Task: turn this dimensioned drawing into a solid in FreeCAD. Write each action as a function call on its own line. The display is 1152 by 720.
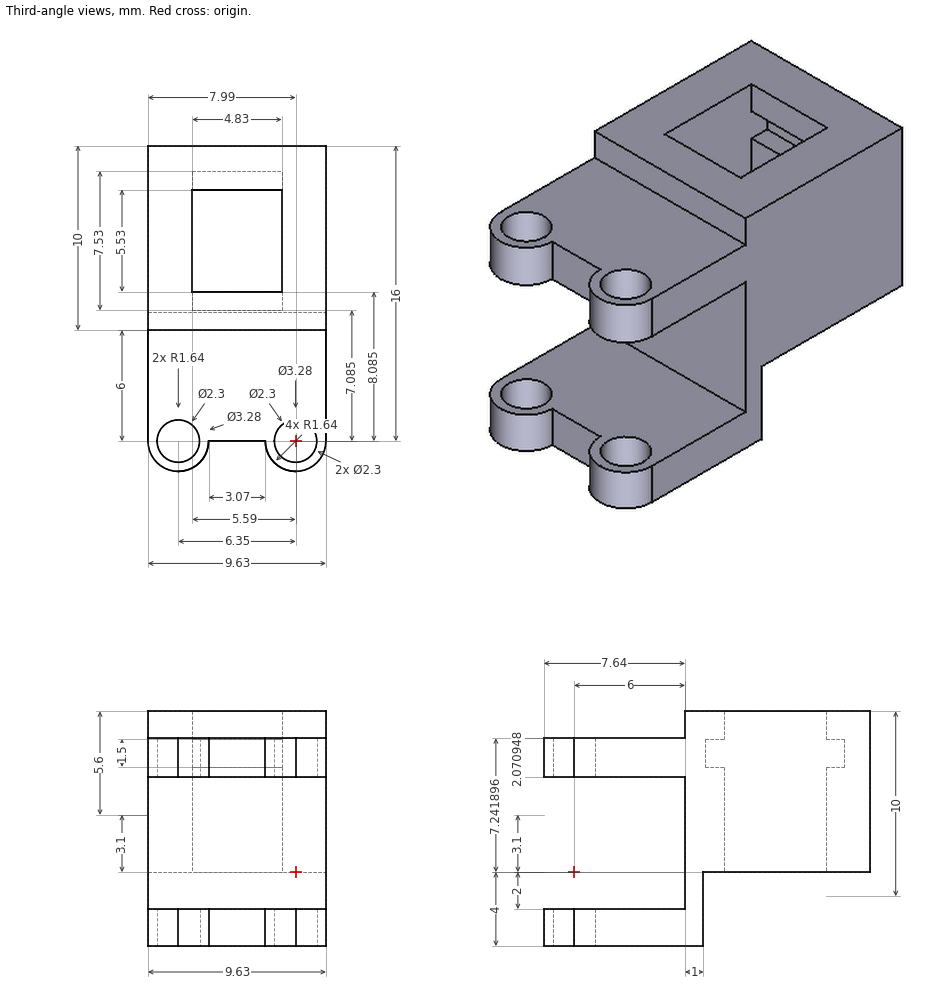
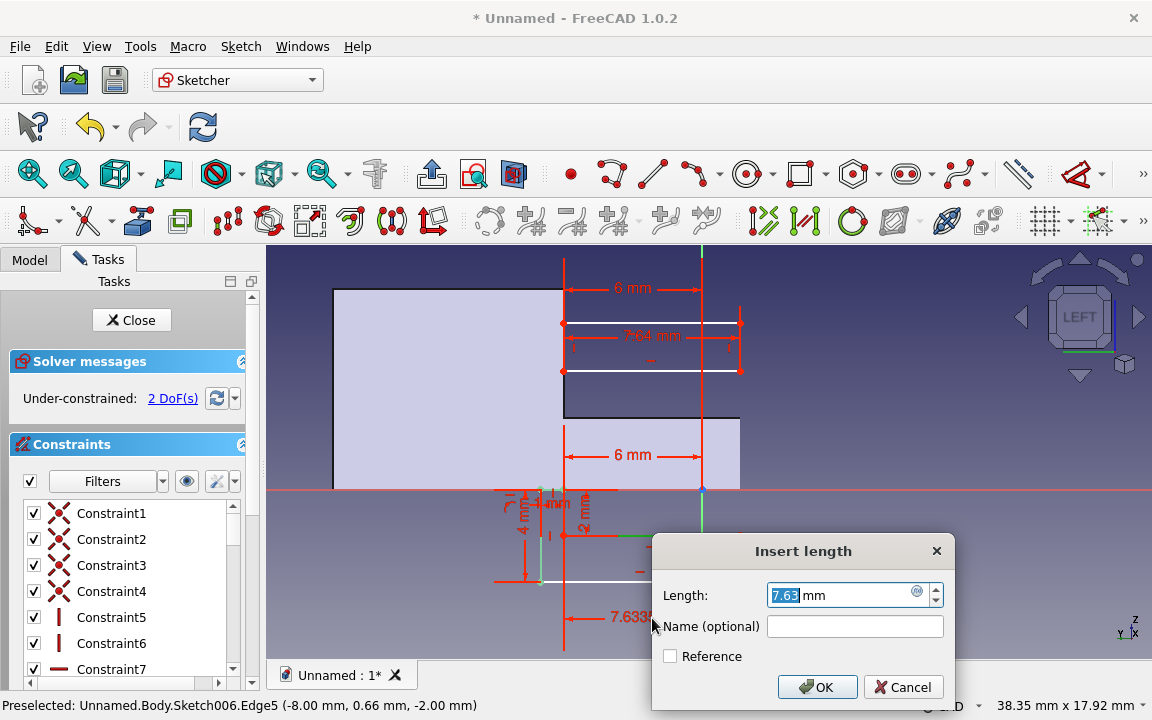
text(7.64)
key(Return)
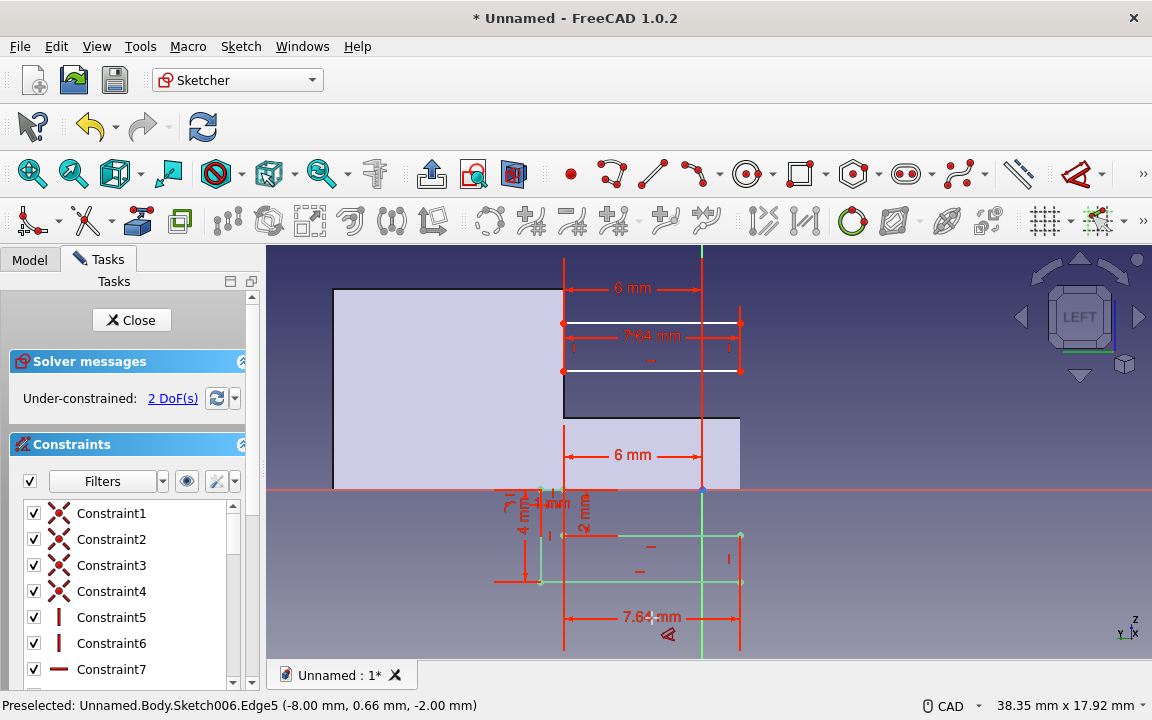
click(564, 337)
click(530, 347)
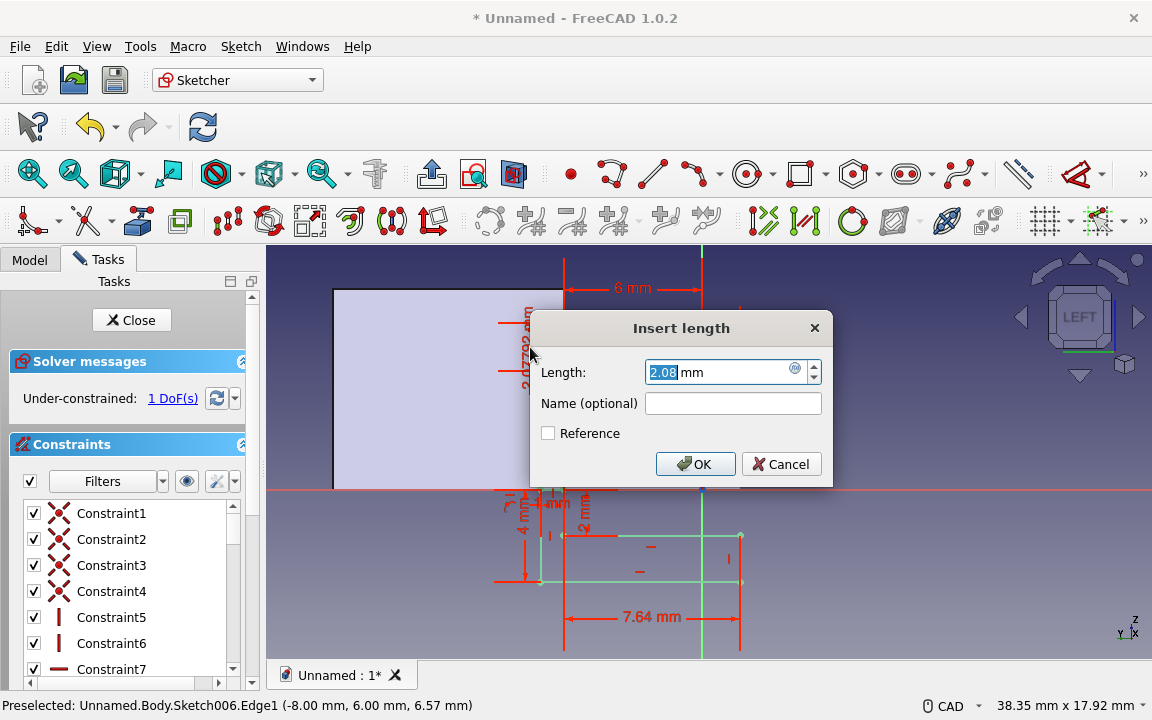
text(2.070948)
key(Return)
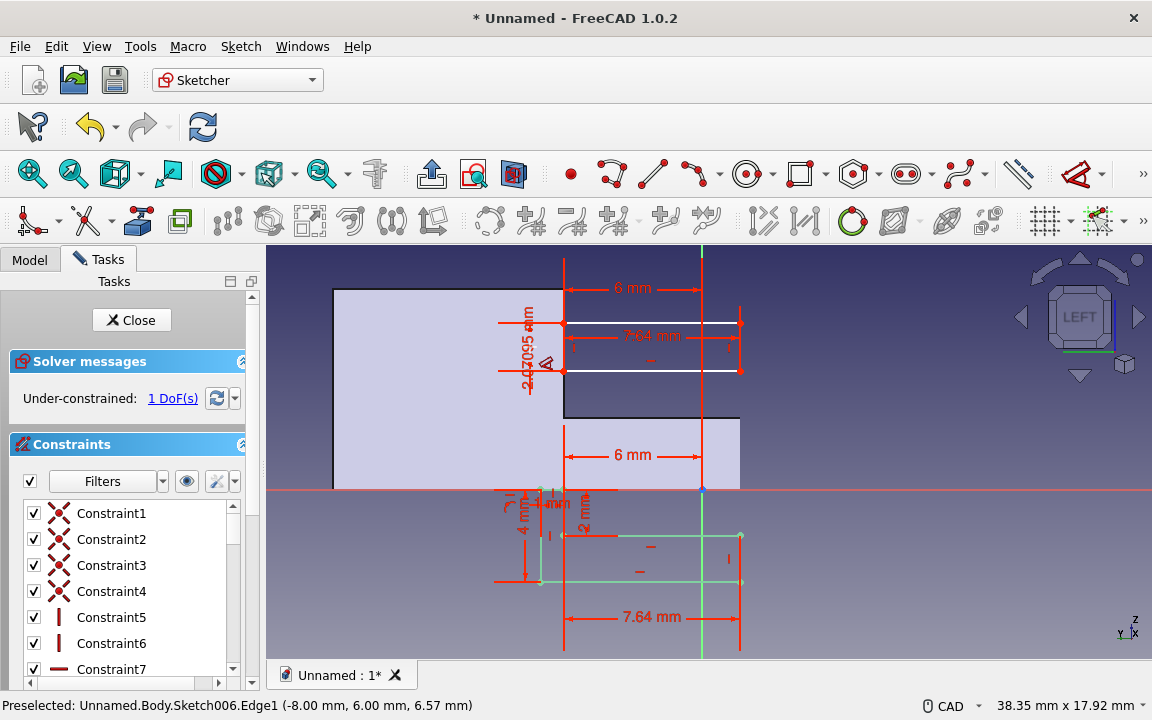
click(564, 323)
click(530, 406)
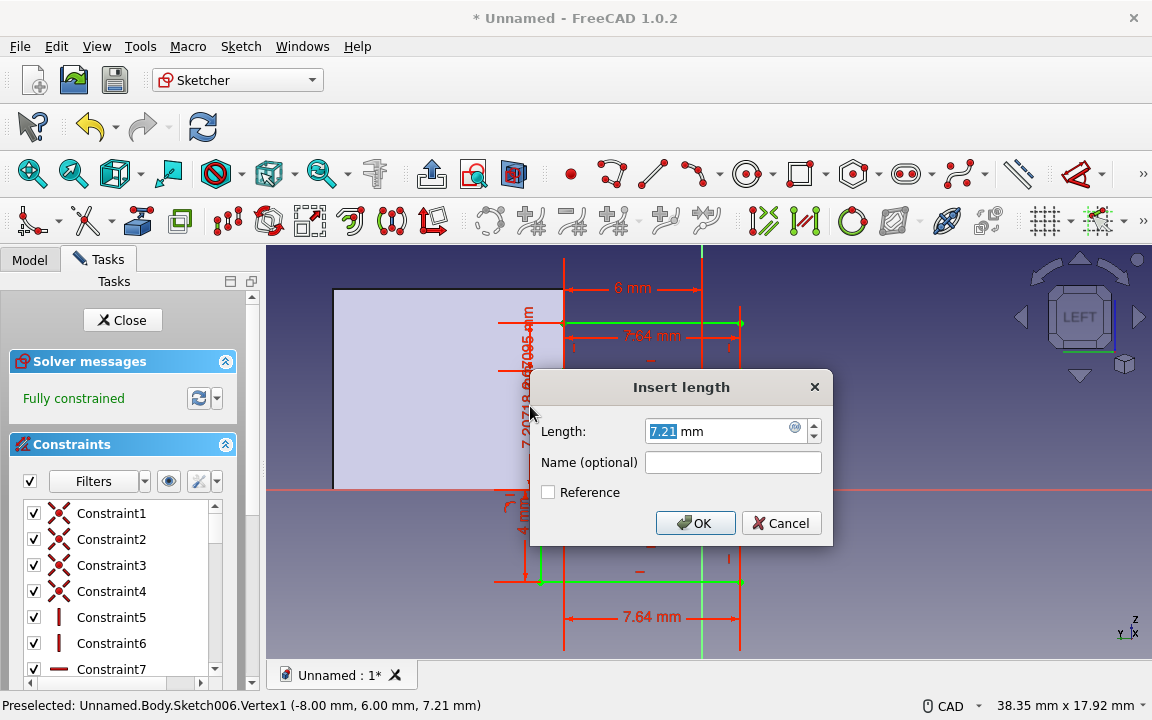
text(7.241896)
key(Return)
key(Escape)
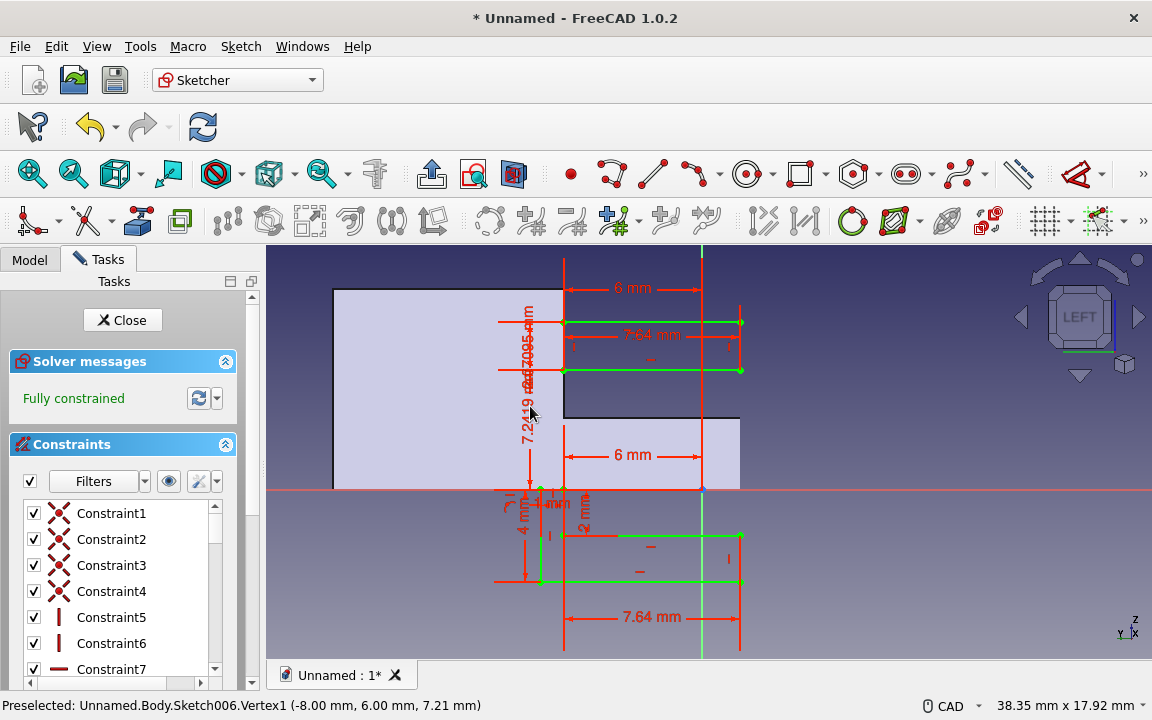
click(123, 320)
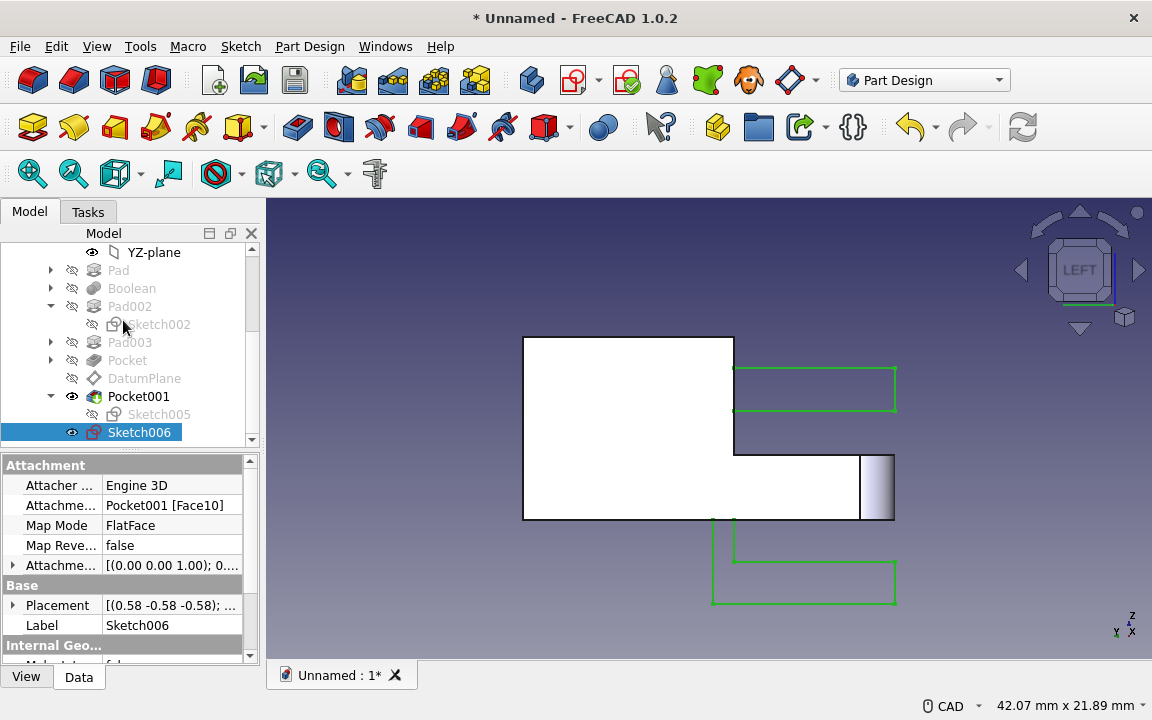
click(33, 128)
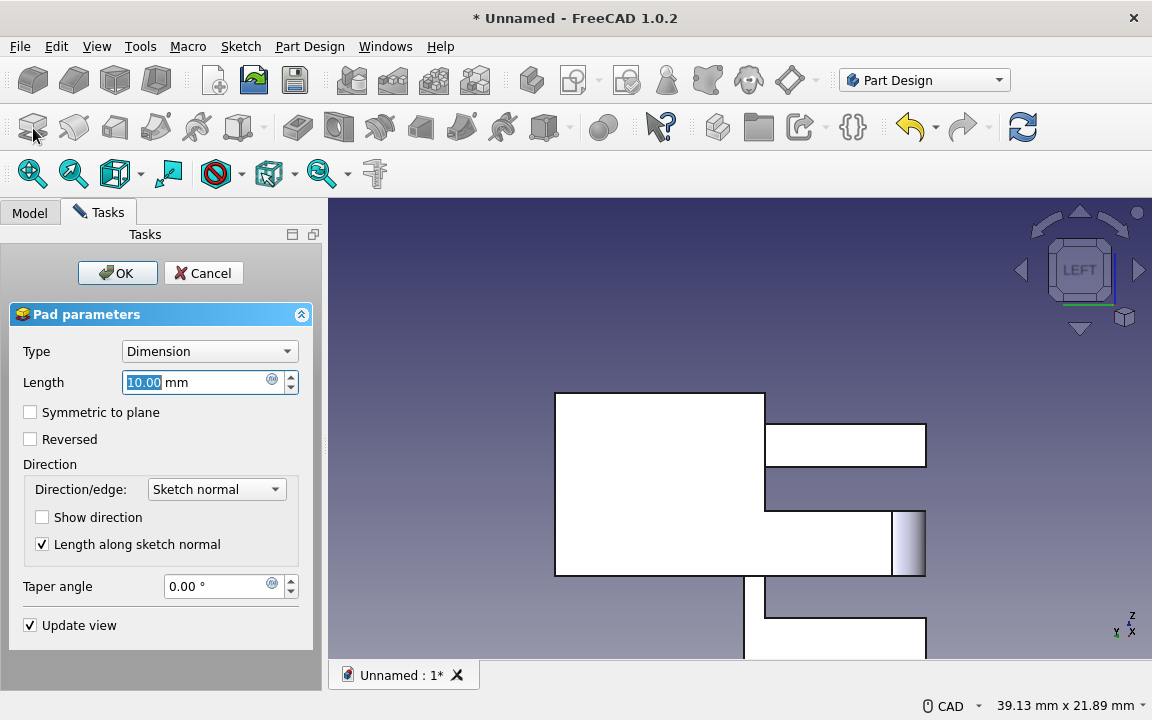
text(9.63)
key(Tab)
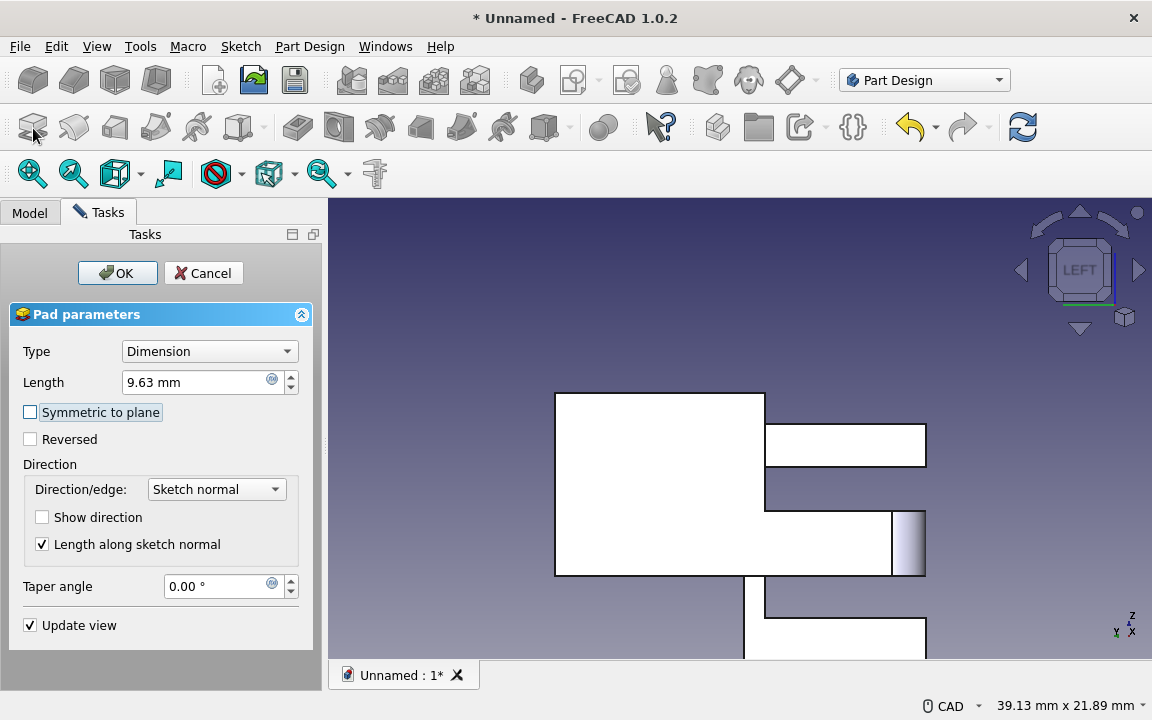
click(31, 439)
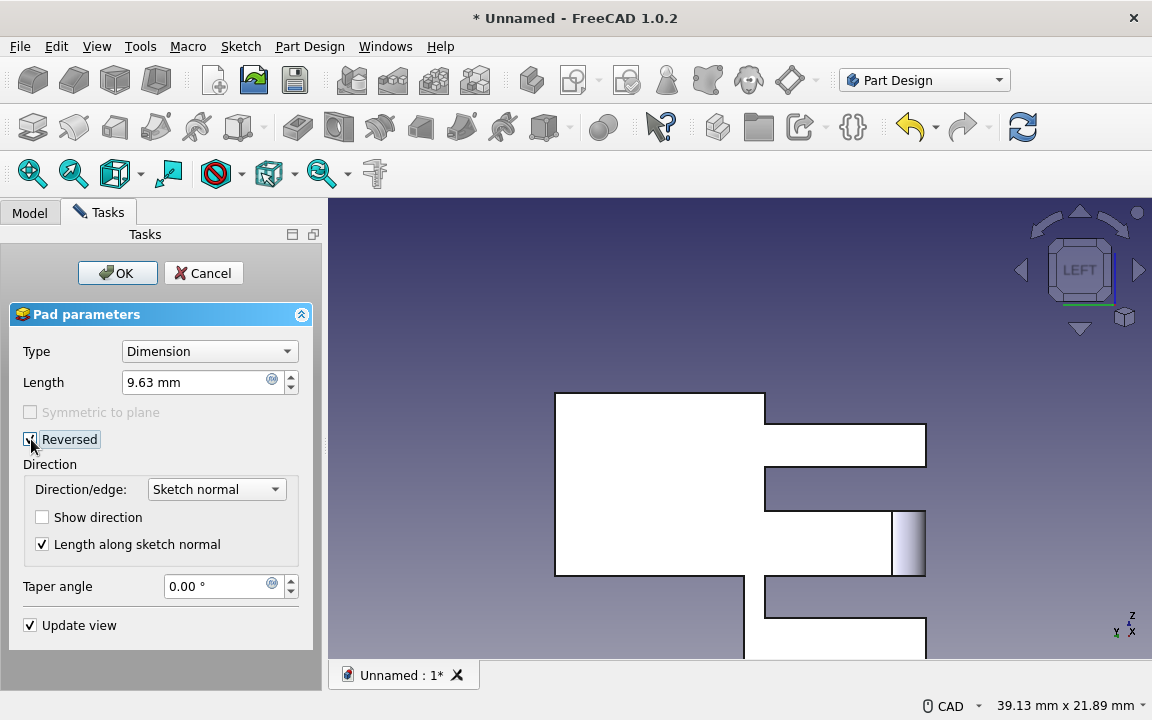
click(118, 273)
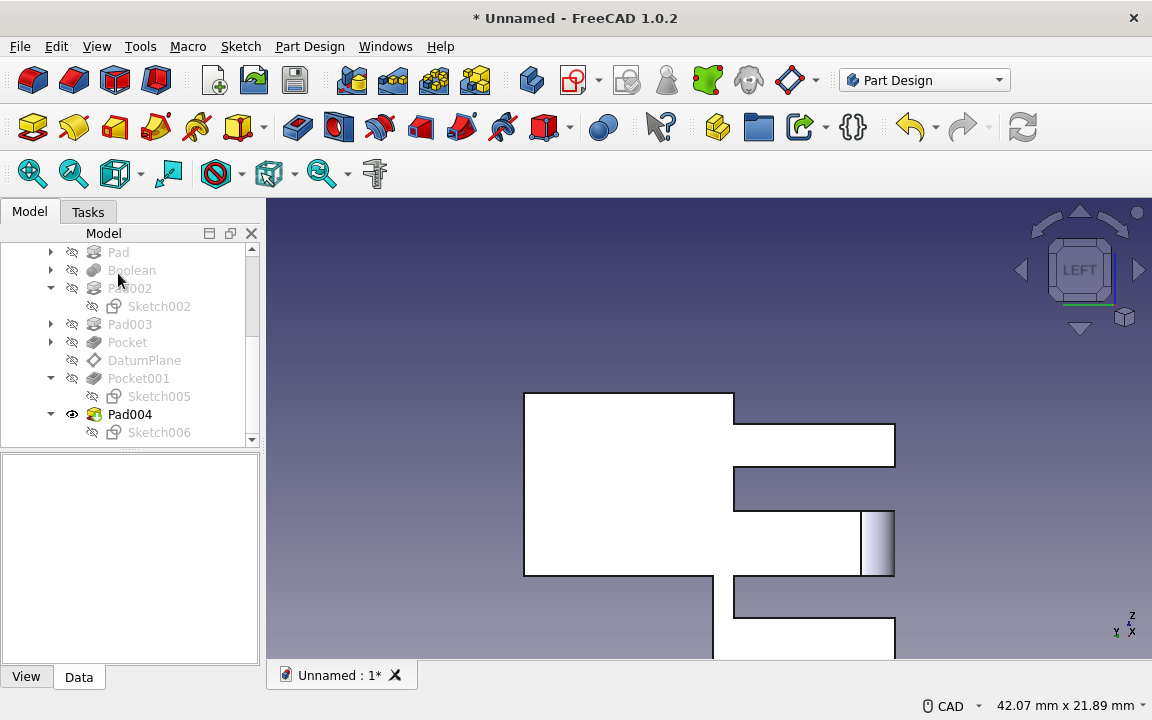
click(33, 174)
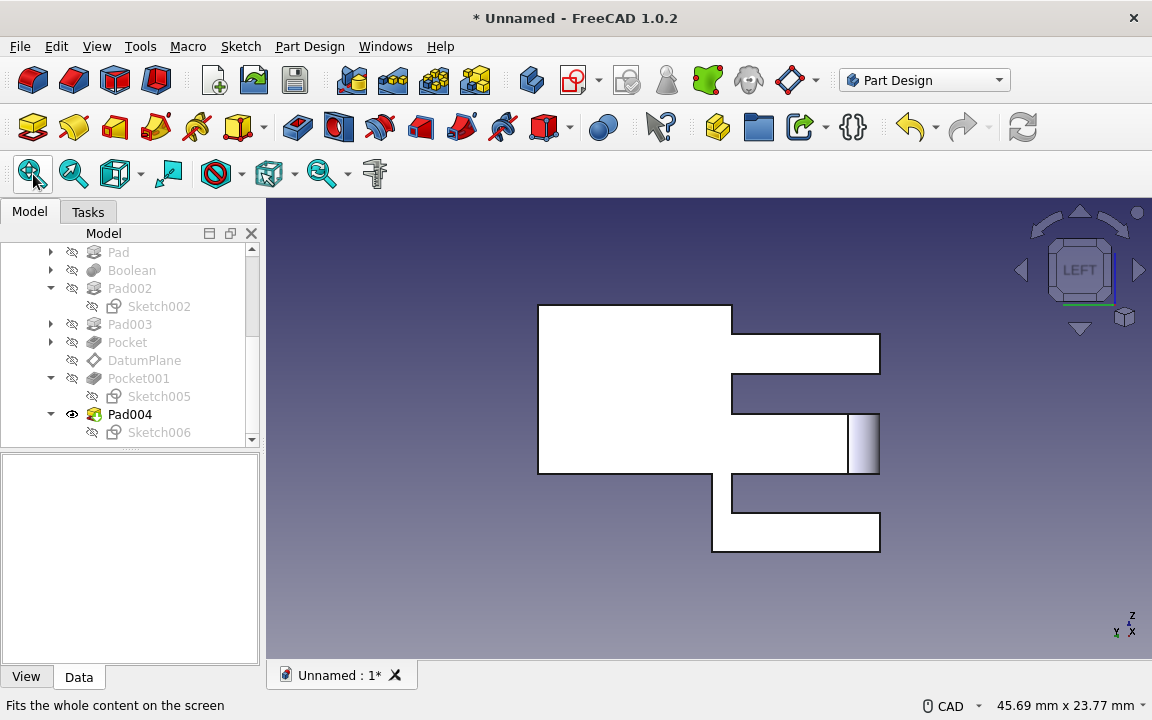
key(5)